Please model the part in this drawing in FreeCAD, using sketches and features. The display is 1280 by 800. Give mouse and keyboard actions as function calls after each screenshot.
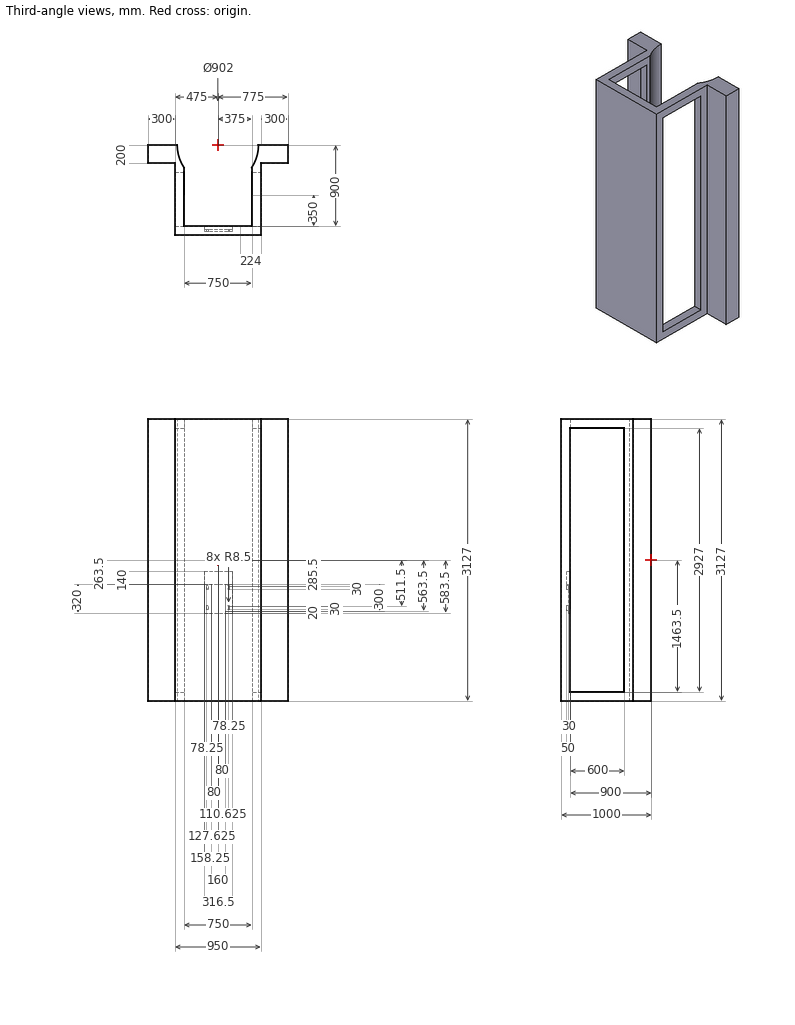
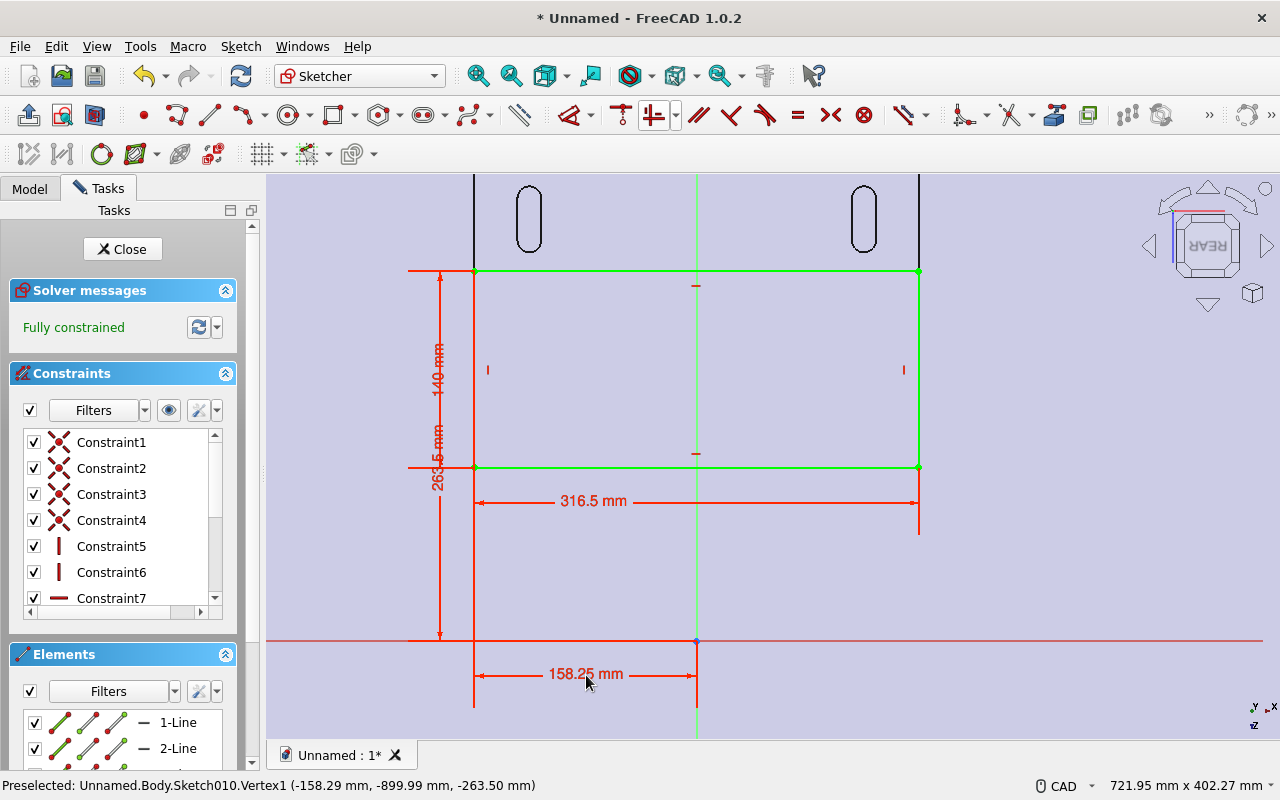
click(123, 249)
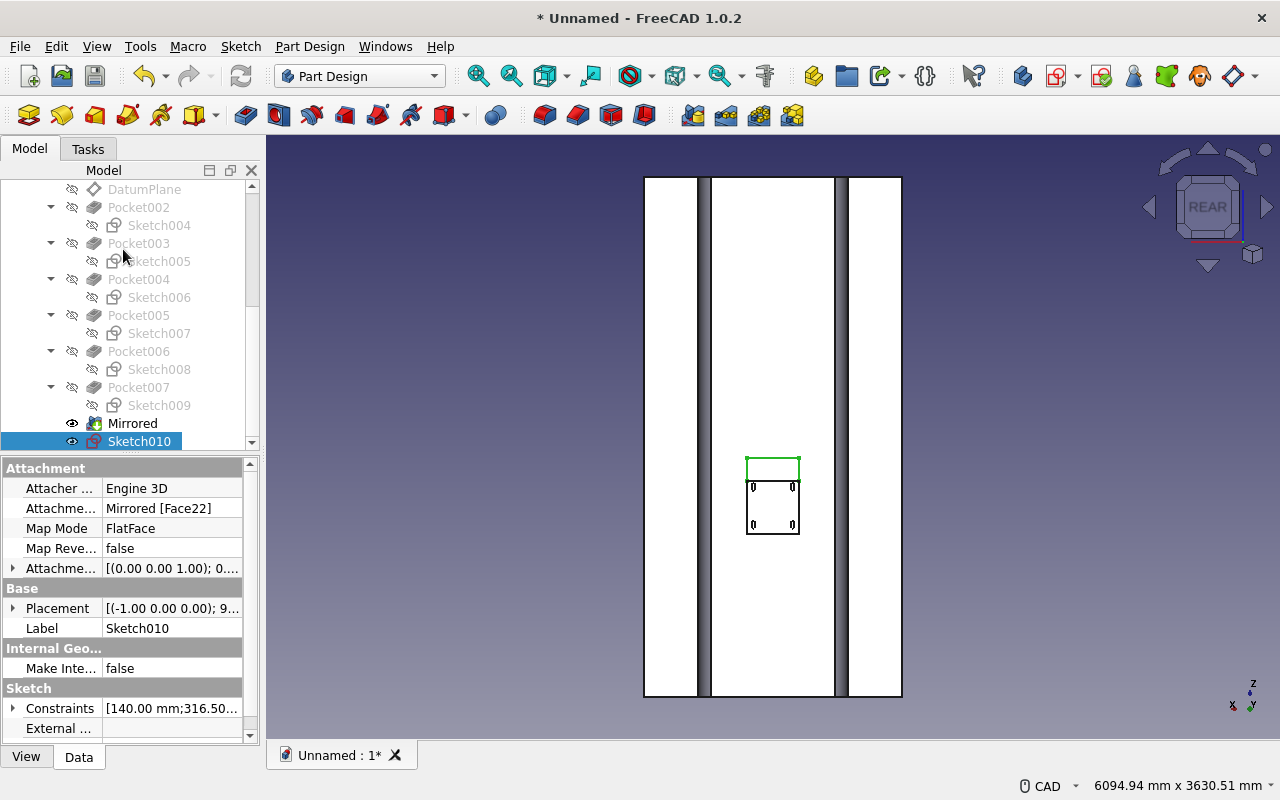
click(246, 116)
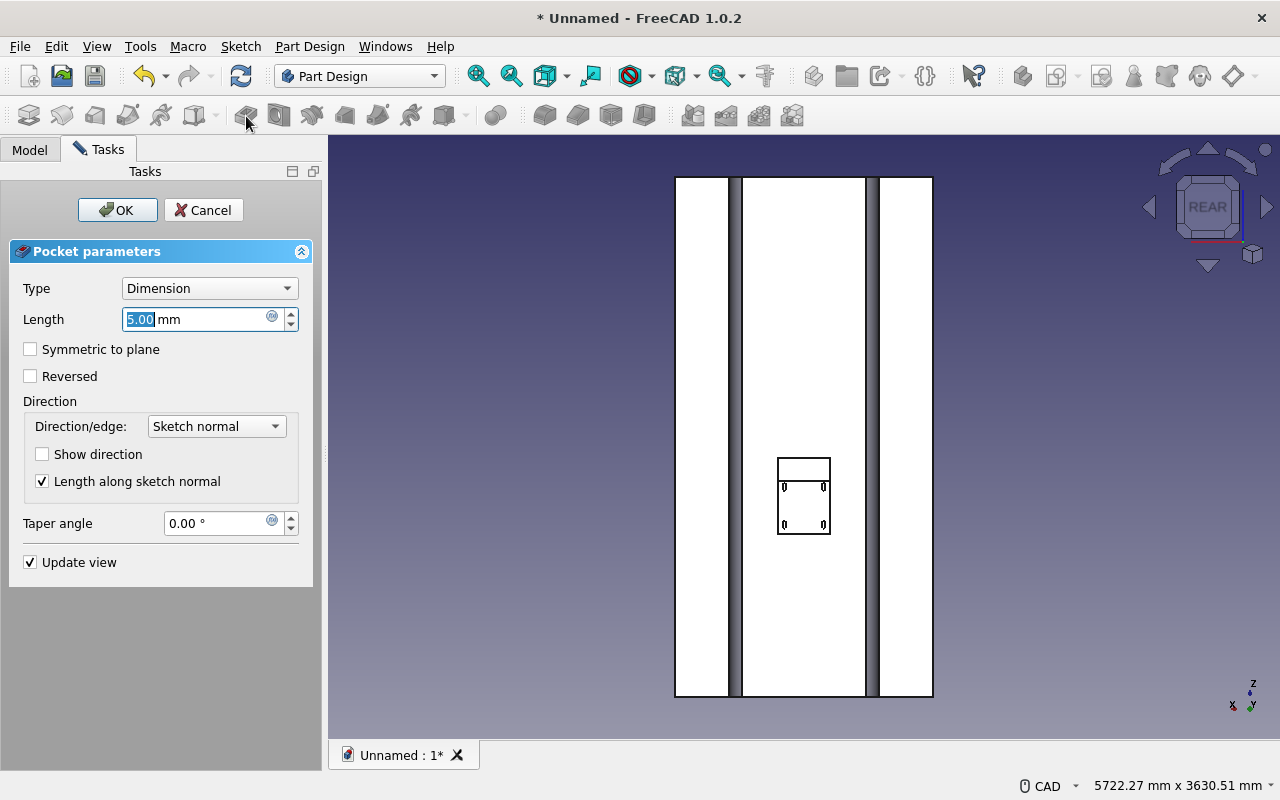
text(50)
key(Tab)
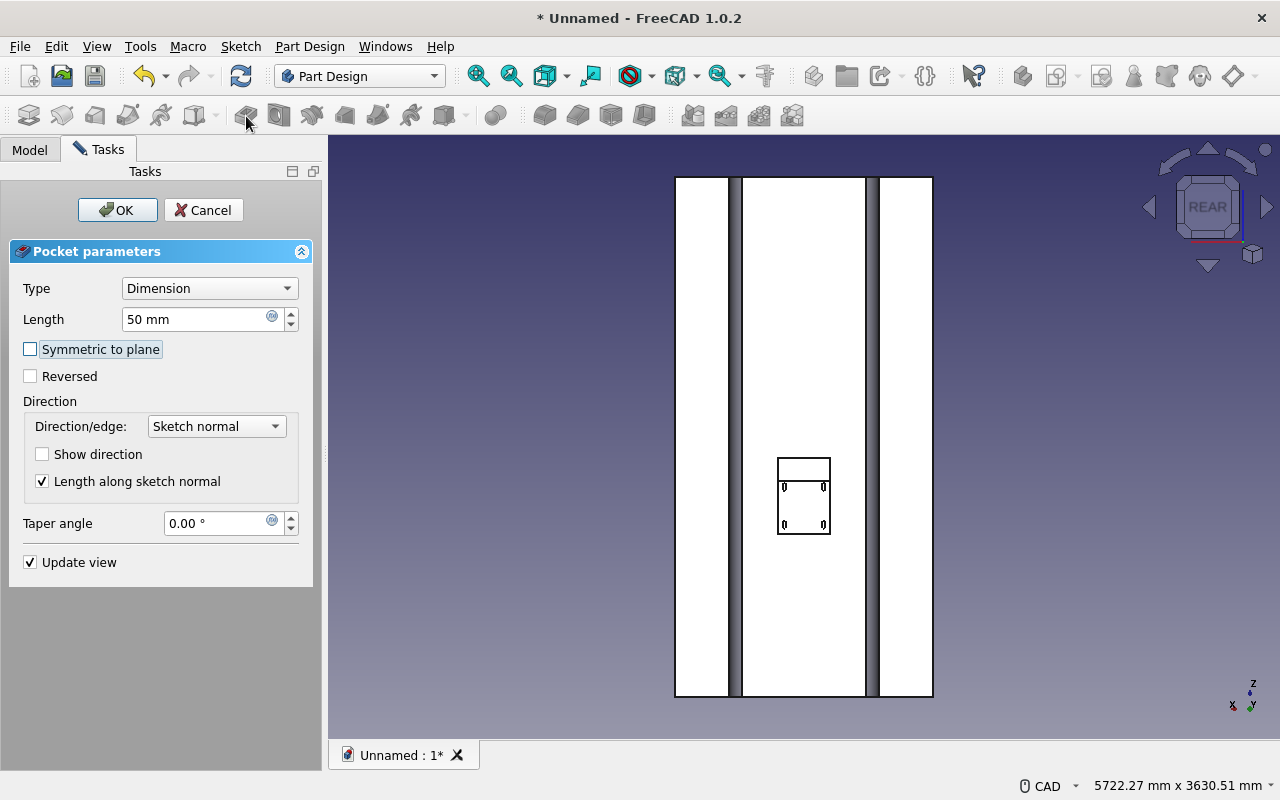
click(118, 210)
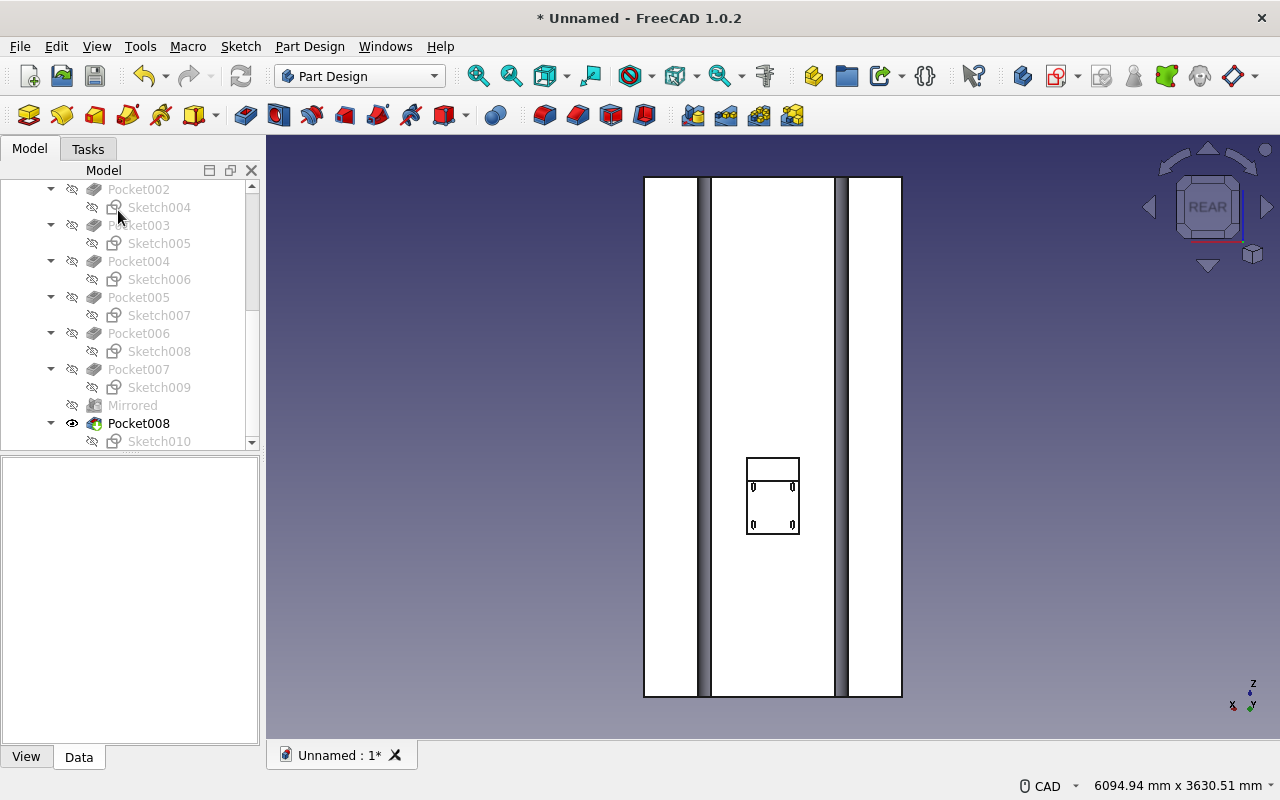
key(0)